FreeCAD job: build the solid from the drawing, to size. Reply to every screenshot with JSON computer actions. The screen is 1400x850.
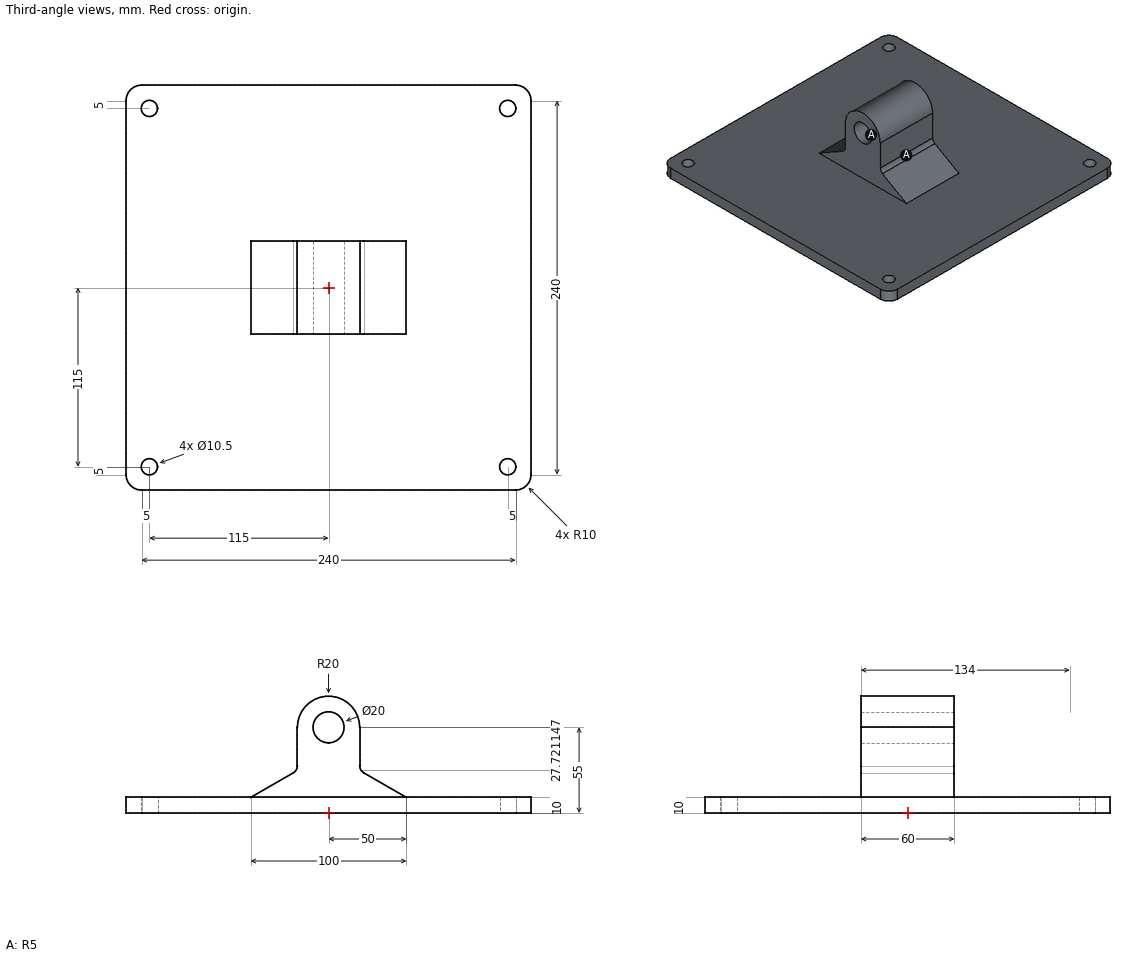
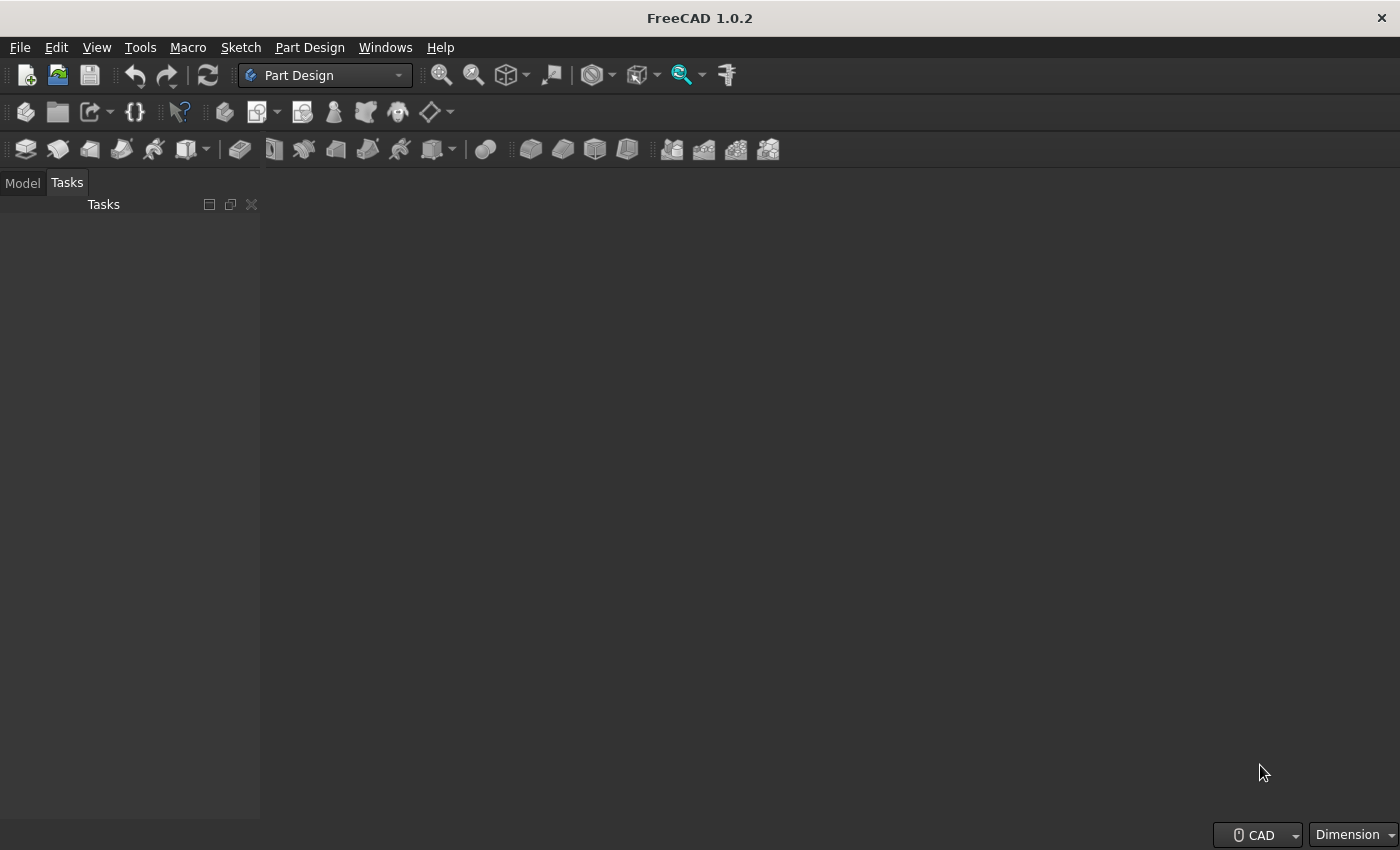
{"action": "left_click", "coordinate": [26, 76]}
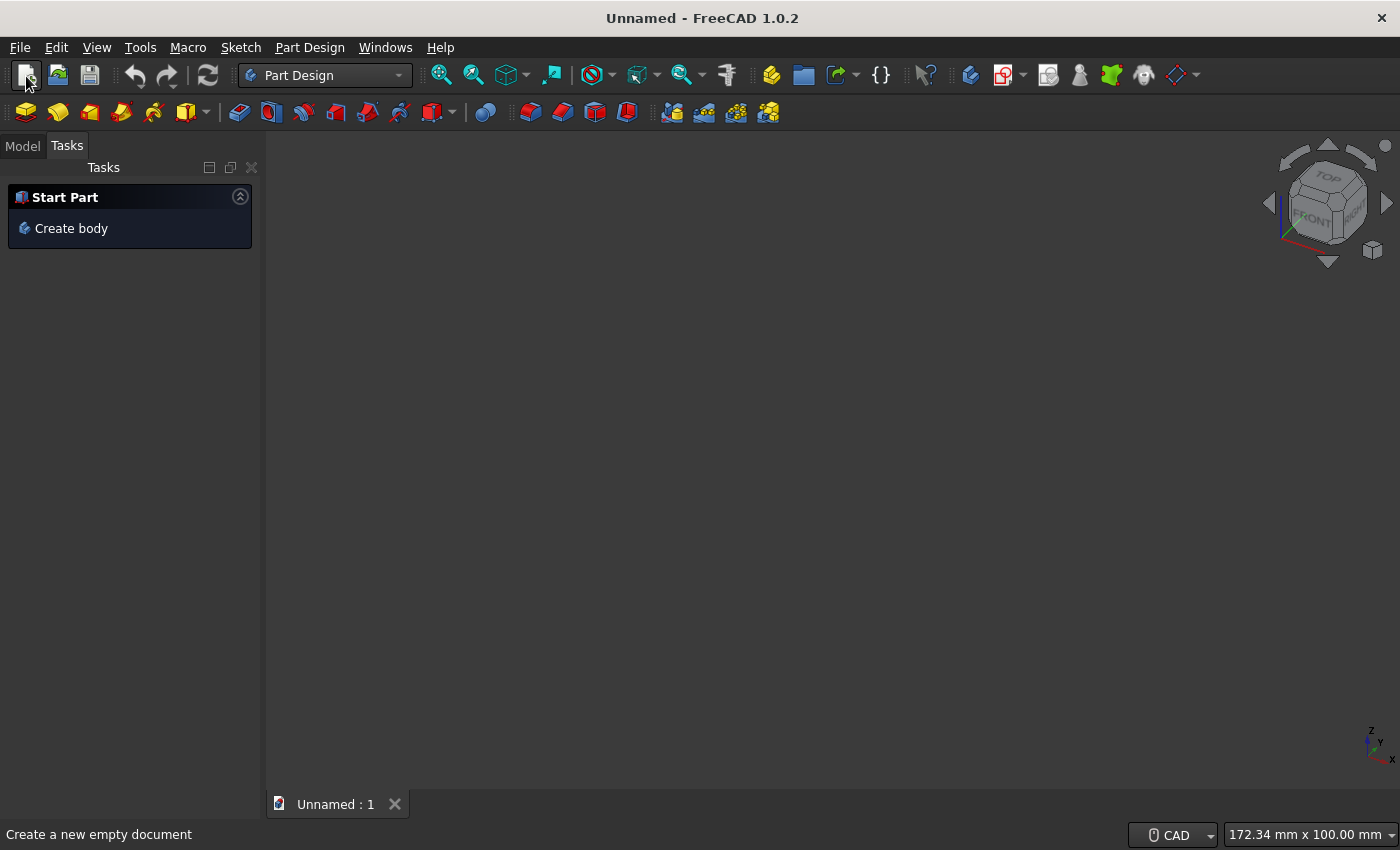
{"action": "left_click", "coordinate": [1004, 76]}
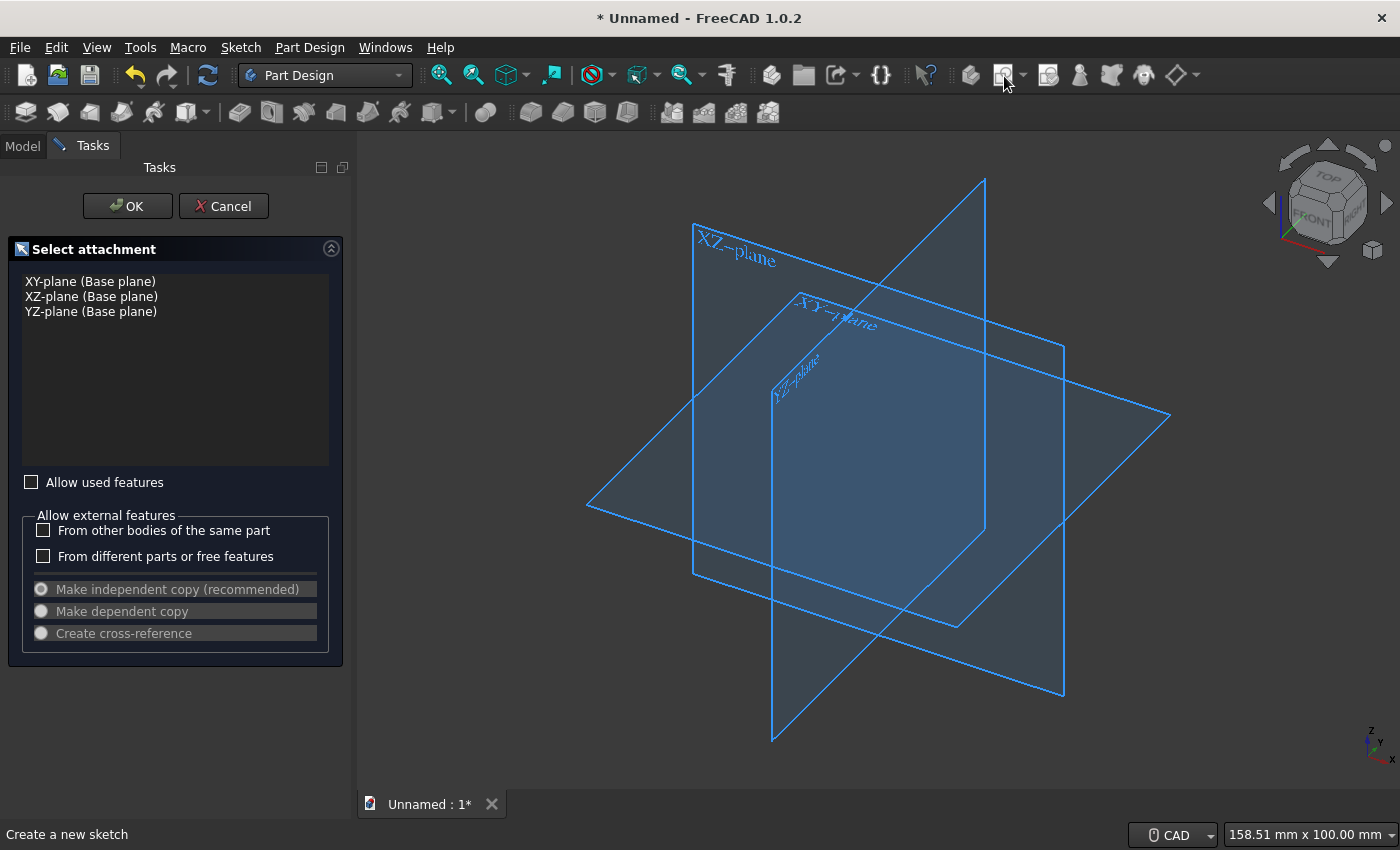
{"action": "left_click", "coordinate": [82, 282]}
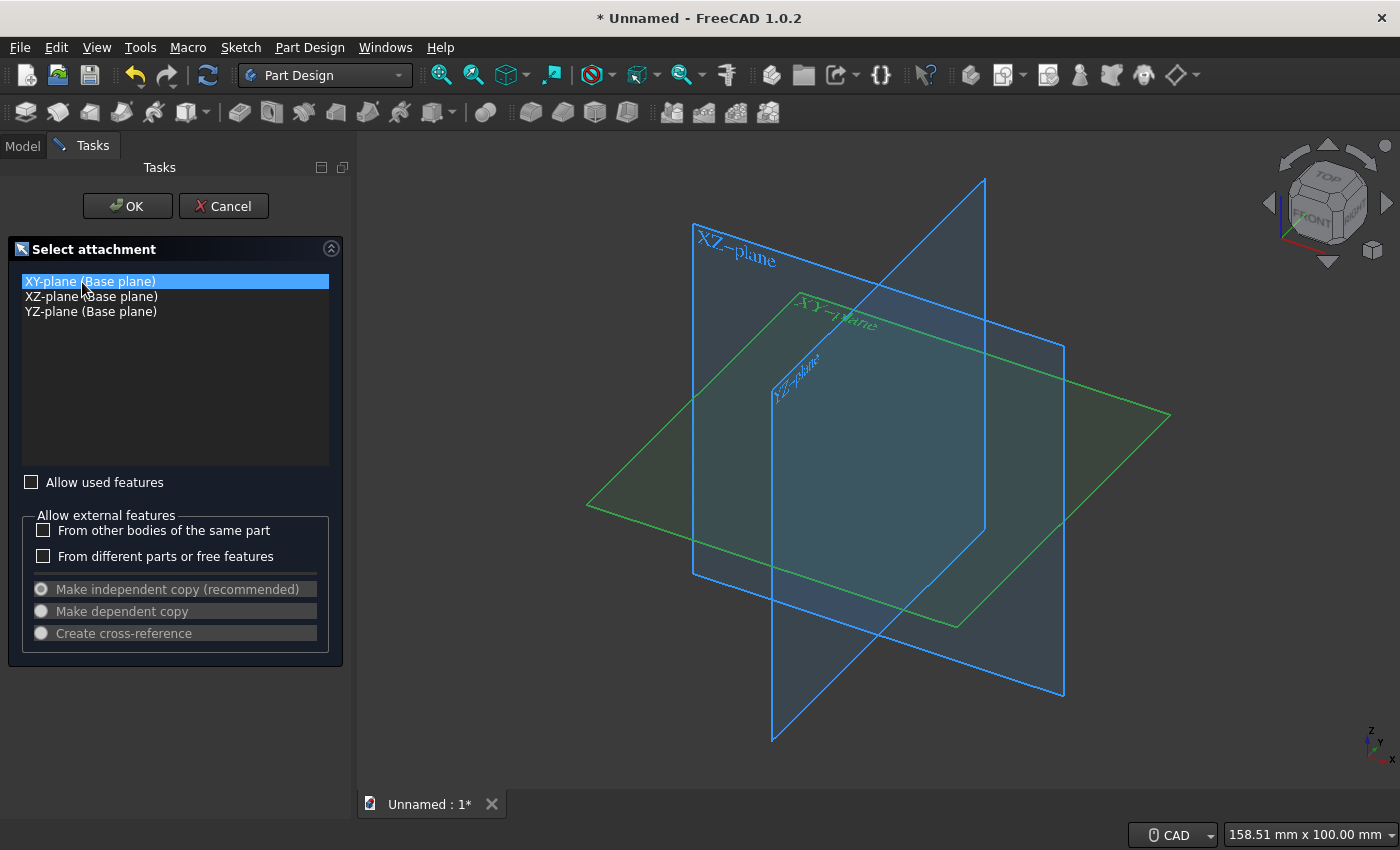
{"action": "left_click", "coordinate": [128, 206]}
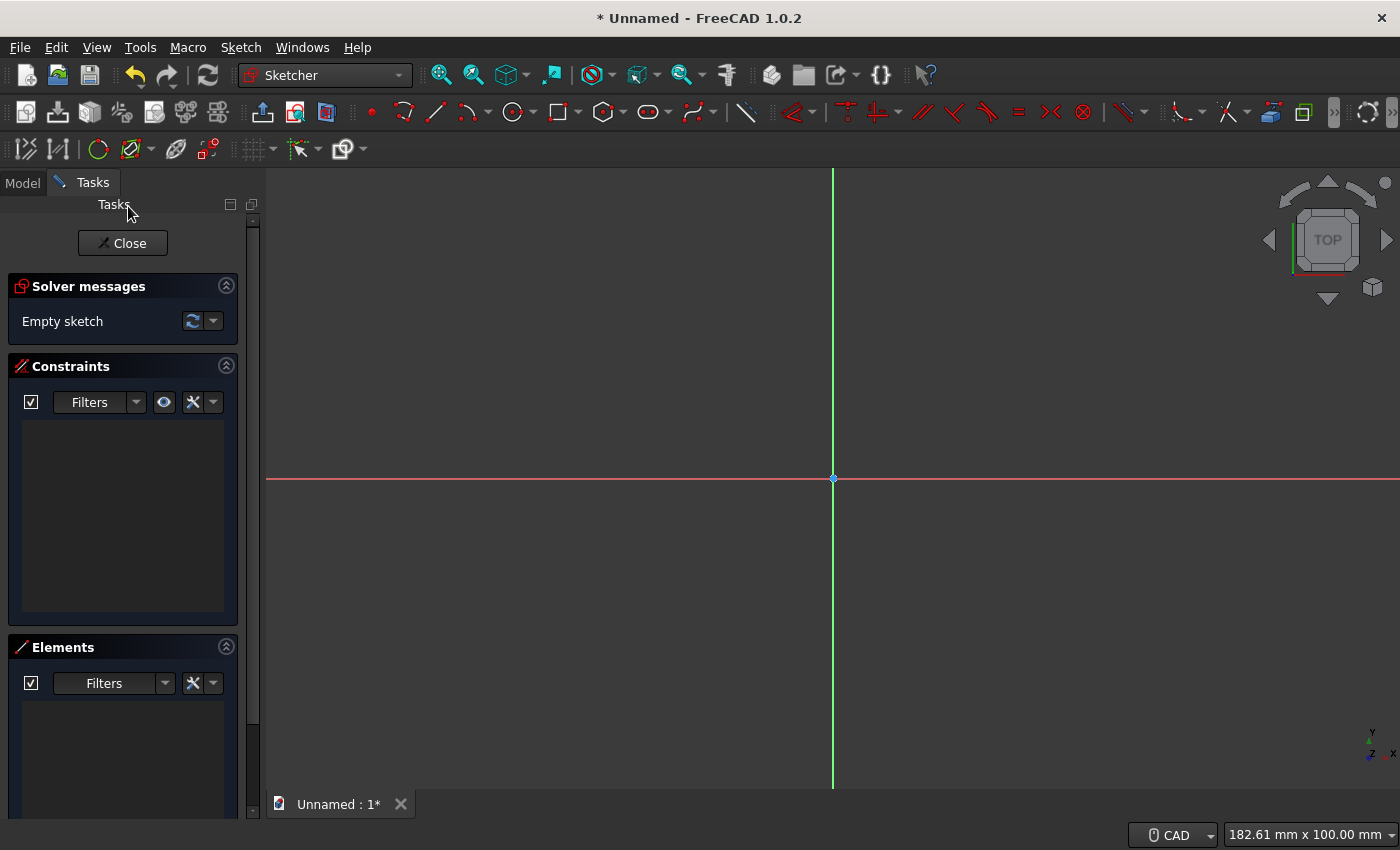
{"action": "scroll", "coordinate": [742, 478], "scroll_direction": "down", "scroll_amount": 7}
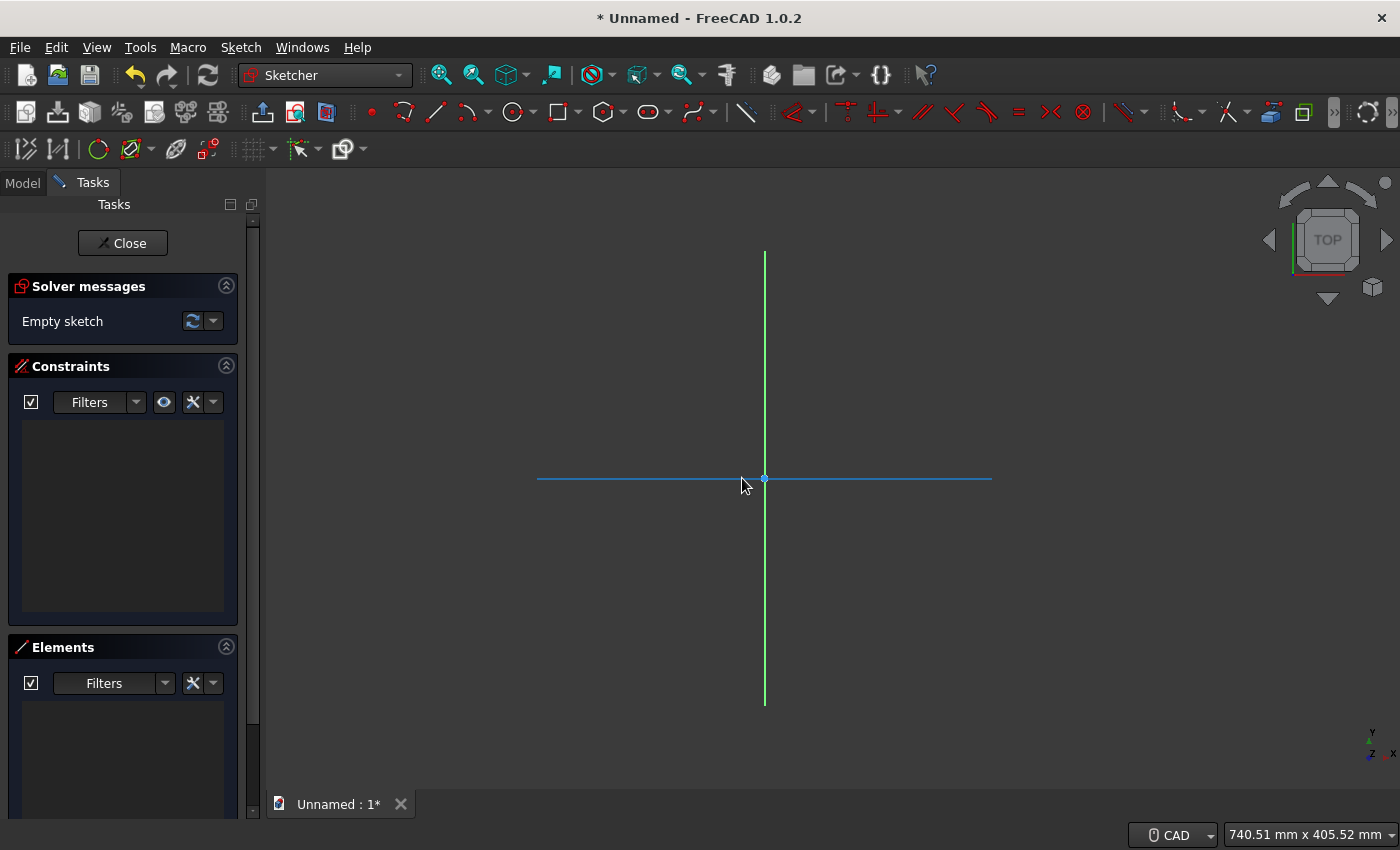
{"action": "left_click", "coordinate": [436, 112]}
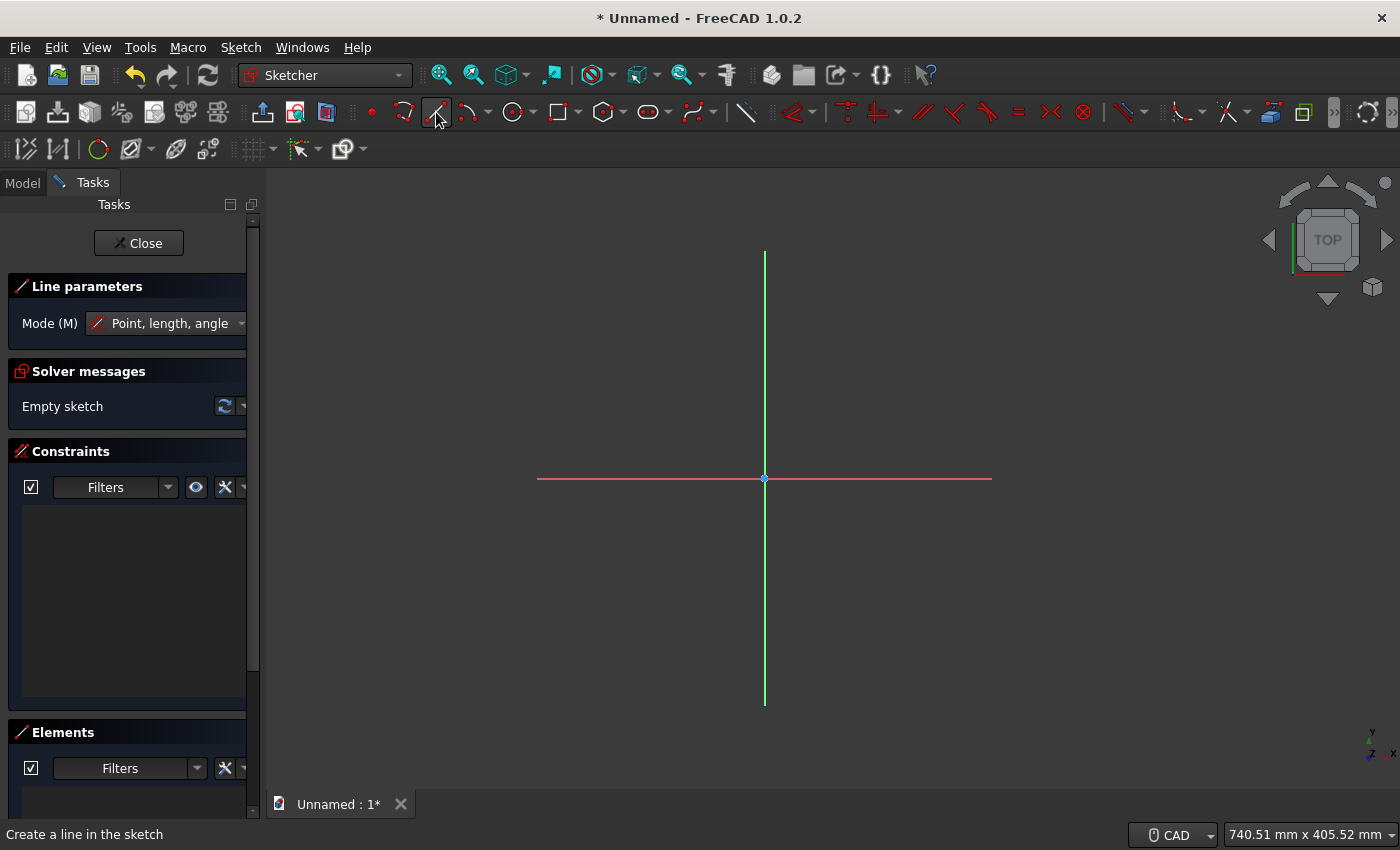
{"action": "left_click", "coordinate": [581, 678]}
{"action": "left_click", "coordinate": [949, 678]}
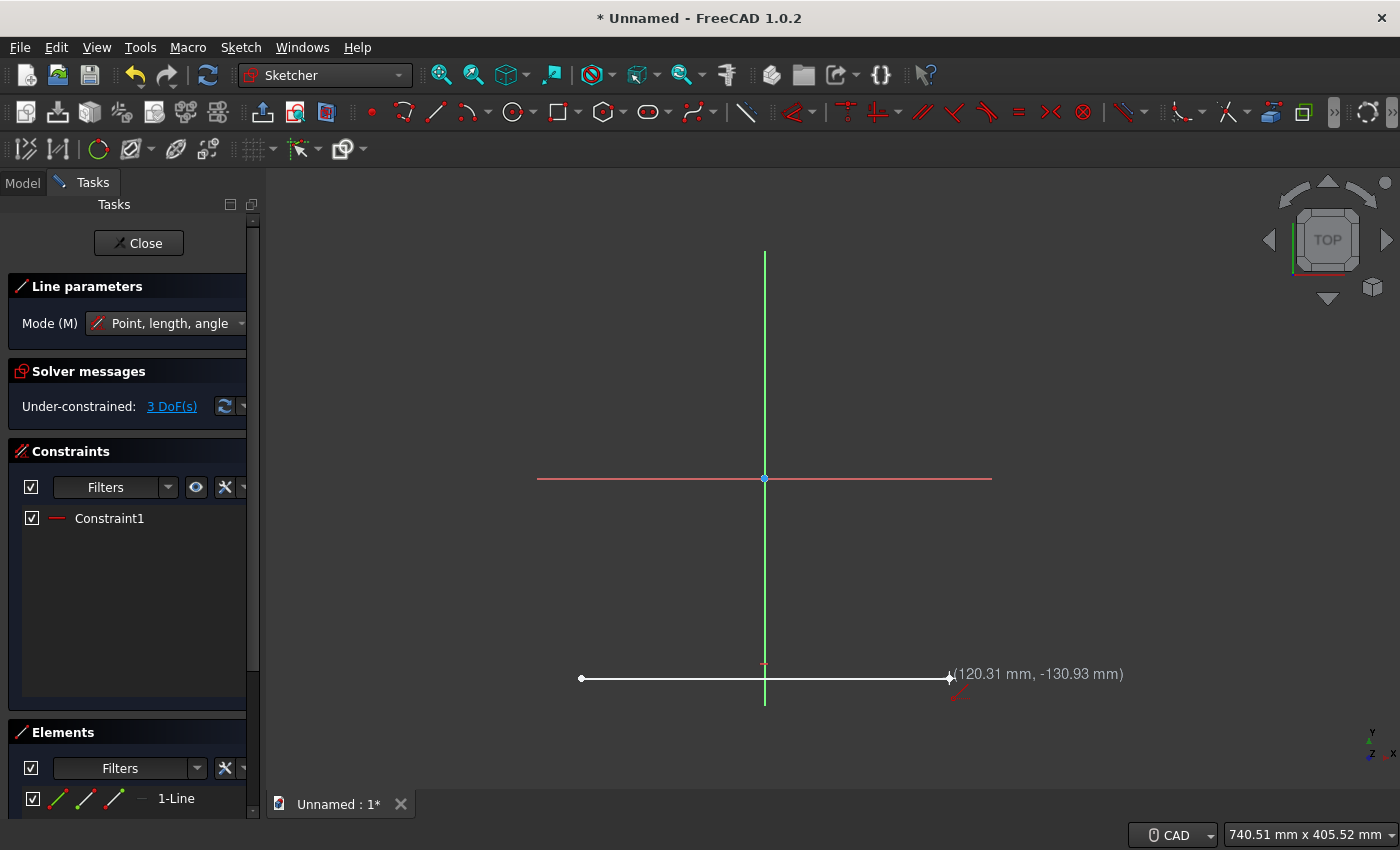
{"action": "left_click", "coordinate": [964, 662]}
{"action": "left_click", "coordinate": [964, 295]}